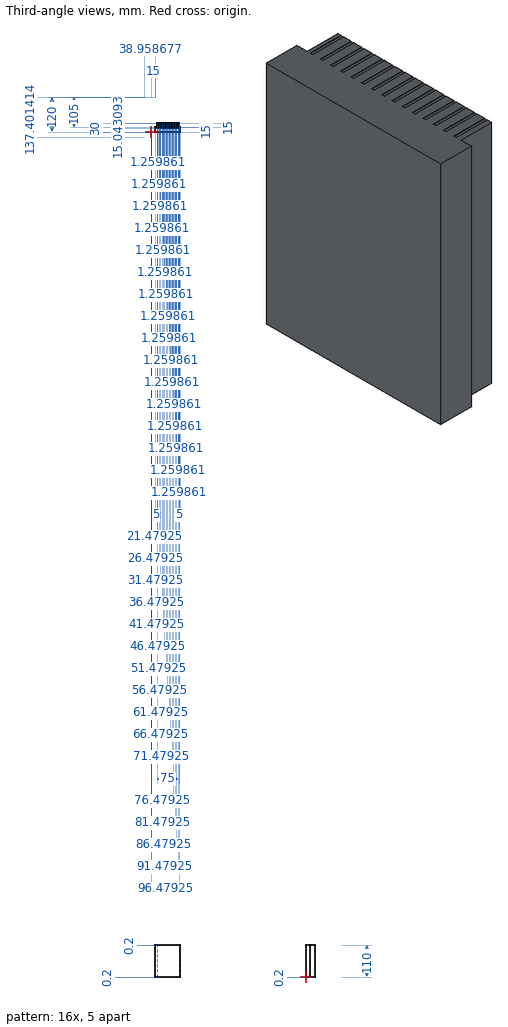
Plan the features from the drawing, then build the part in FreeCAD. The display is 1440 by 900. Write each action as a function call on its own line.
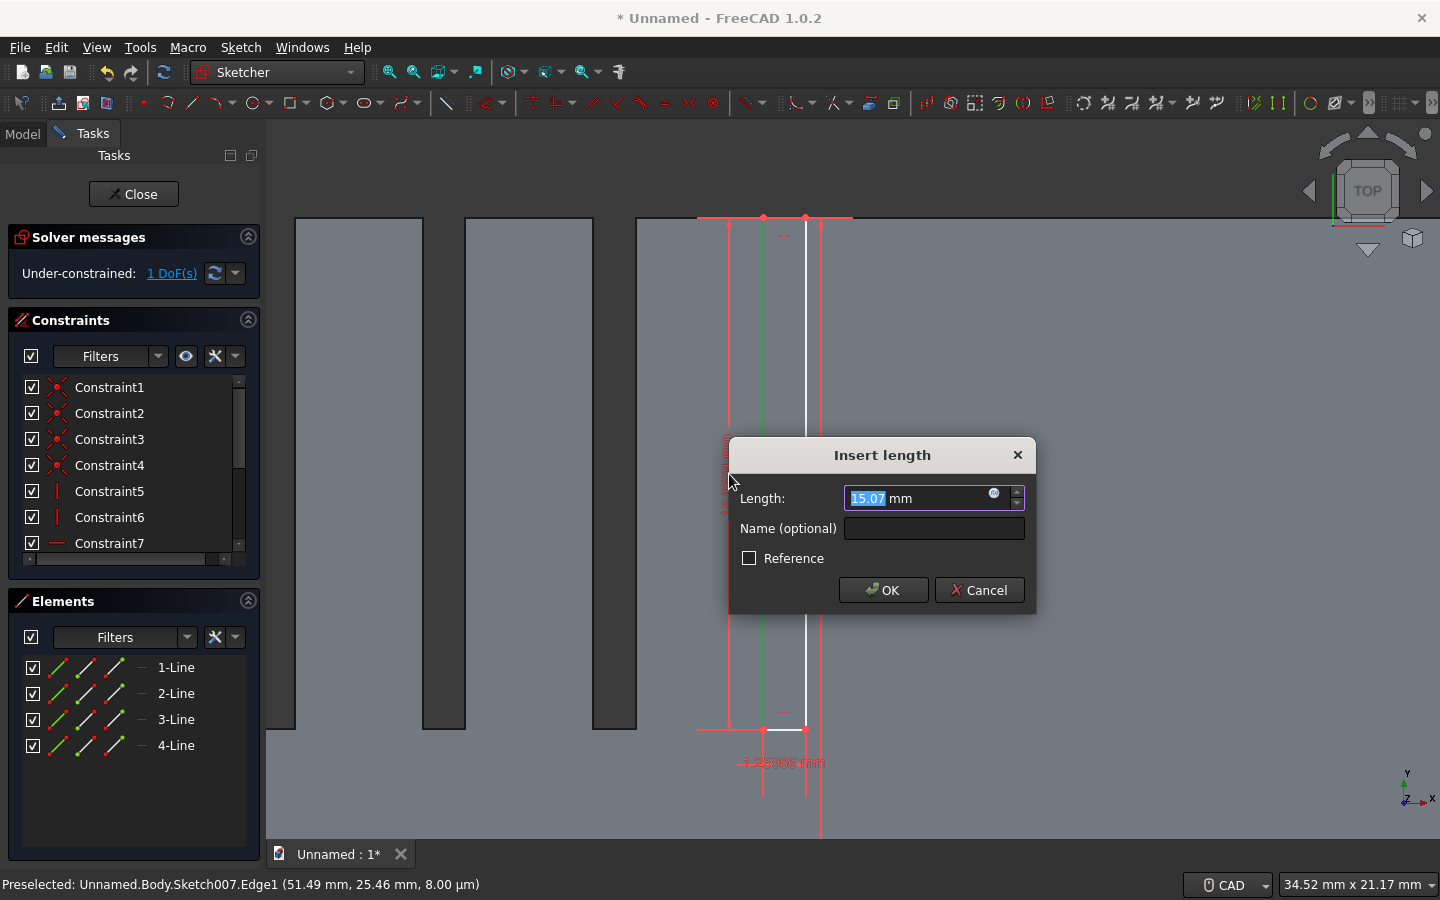
text(15.043093)
key(Return)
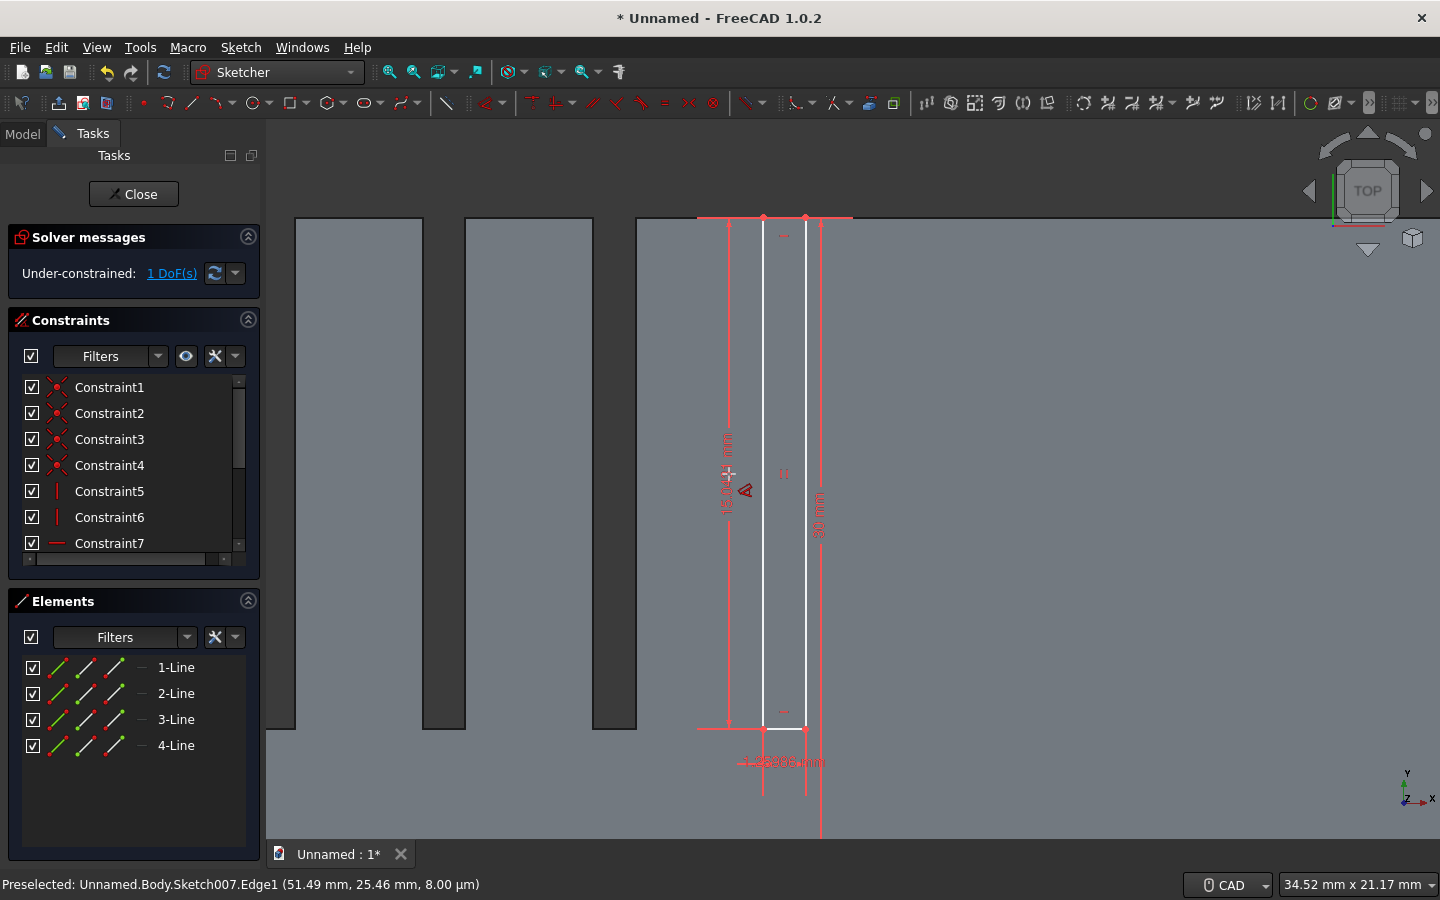
click(763, 218)
click(529, 184)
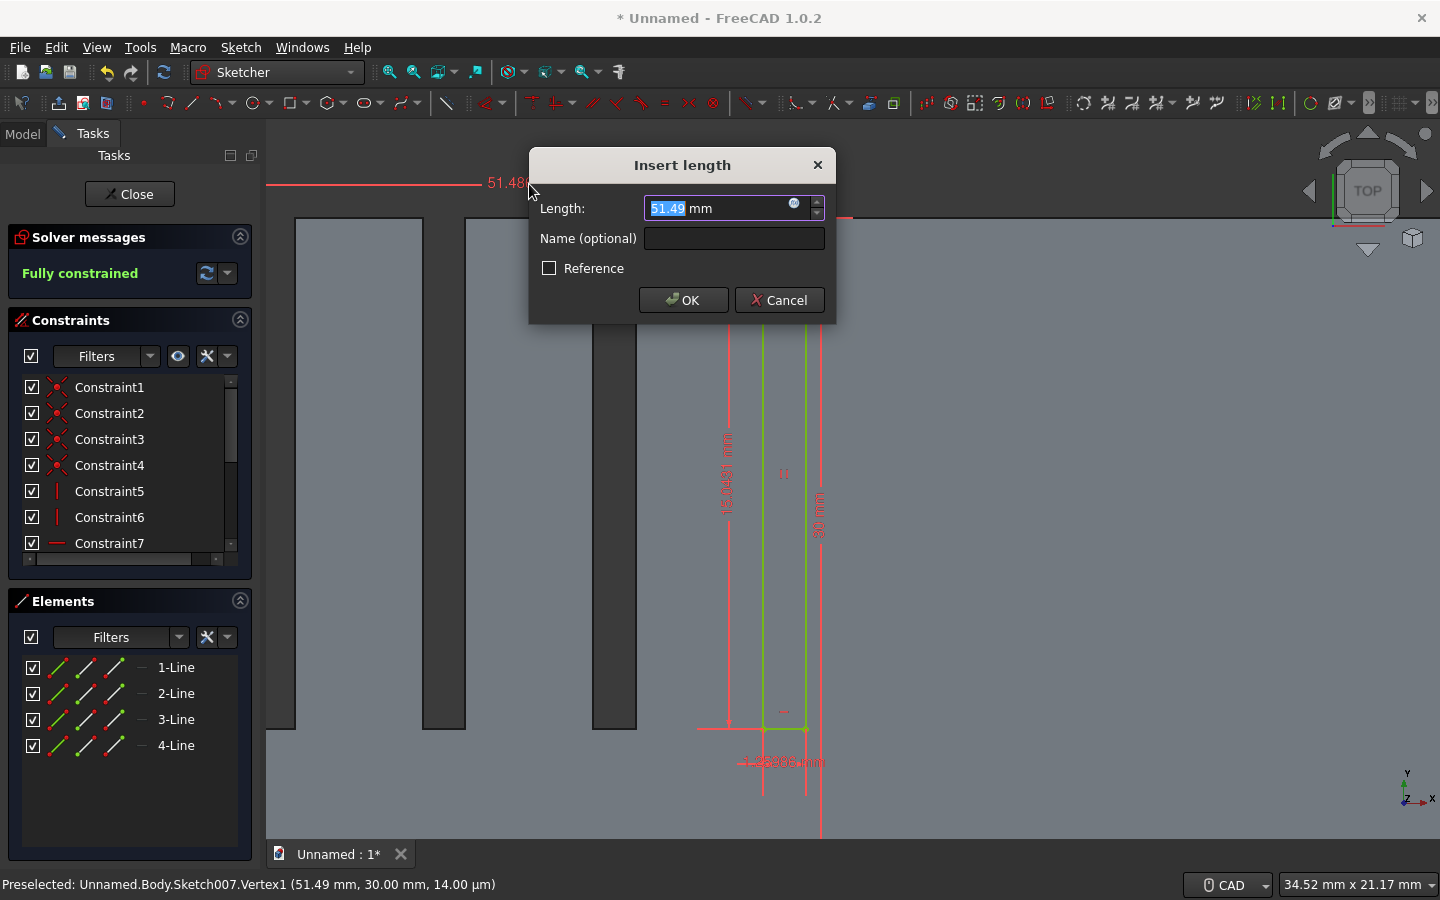
text(51.47925)
key(Return)
key(Escape)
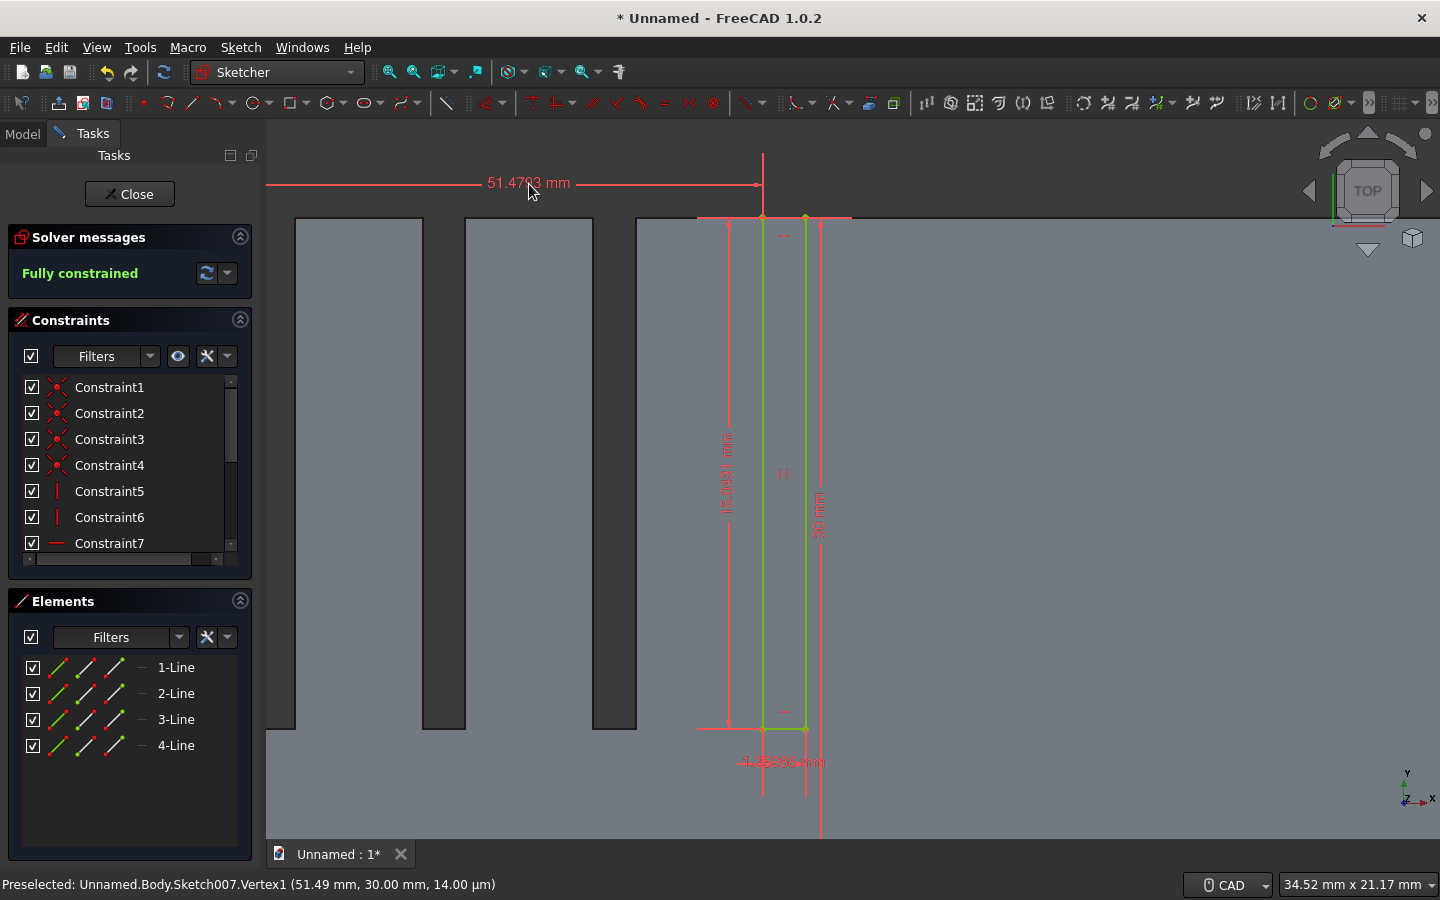
click(130, 194)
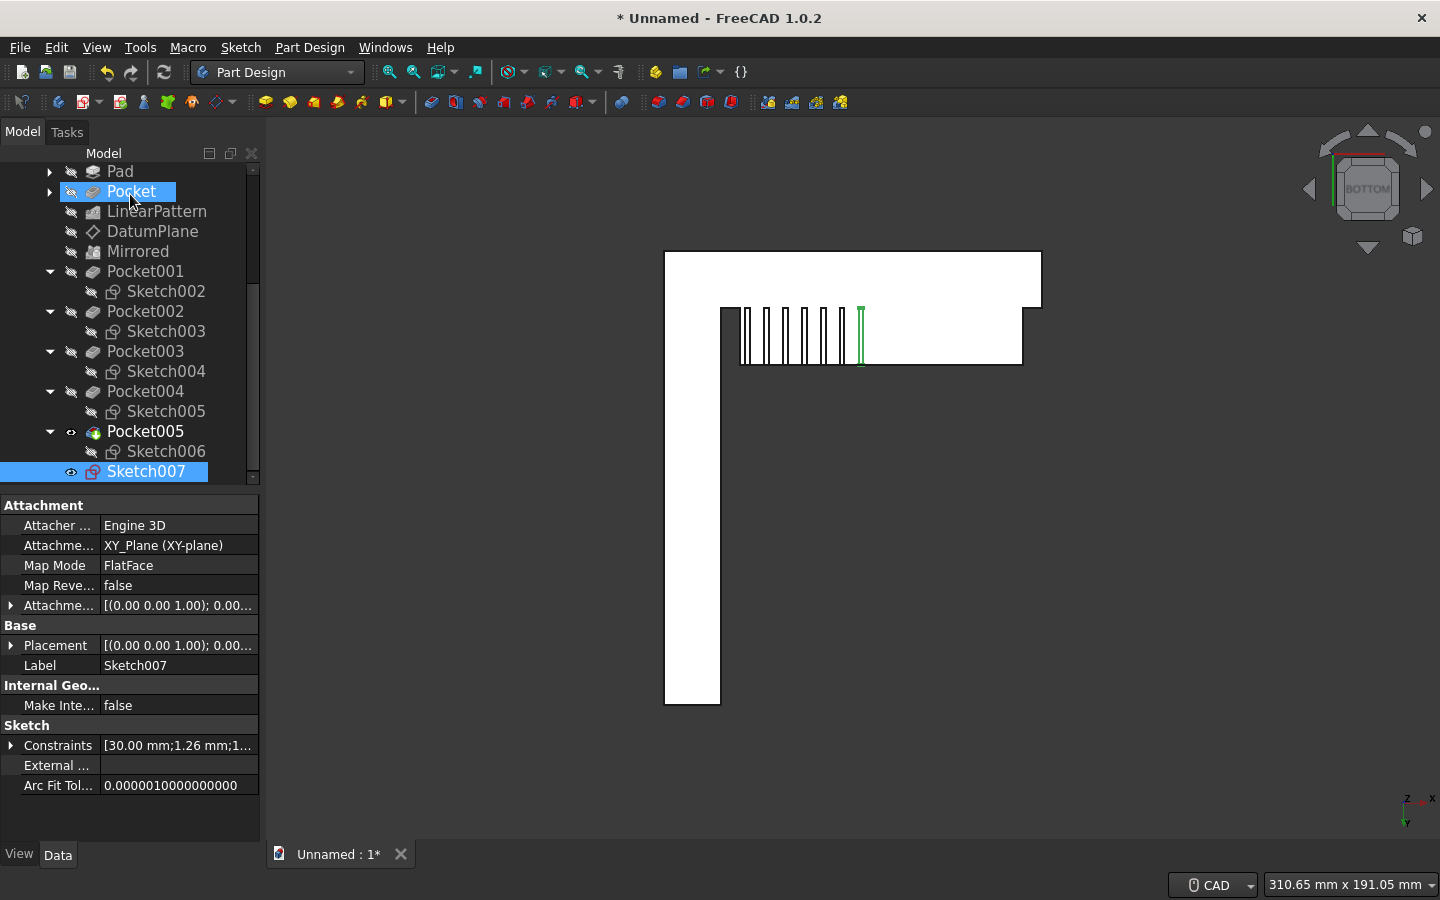
click(432, 102)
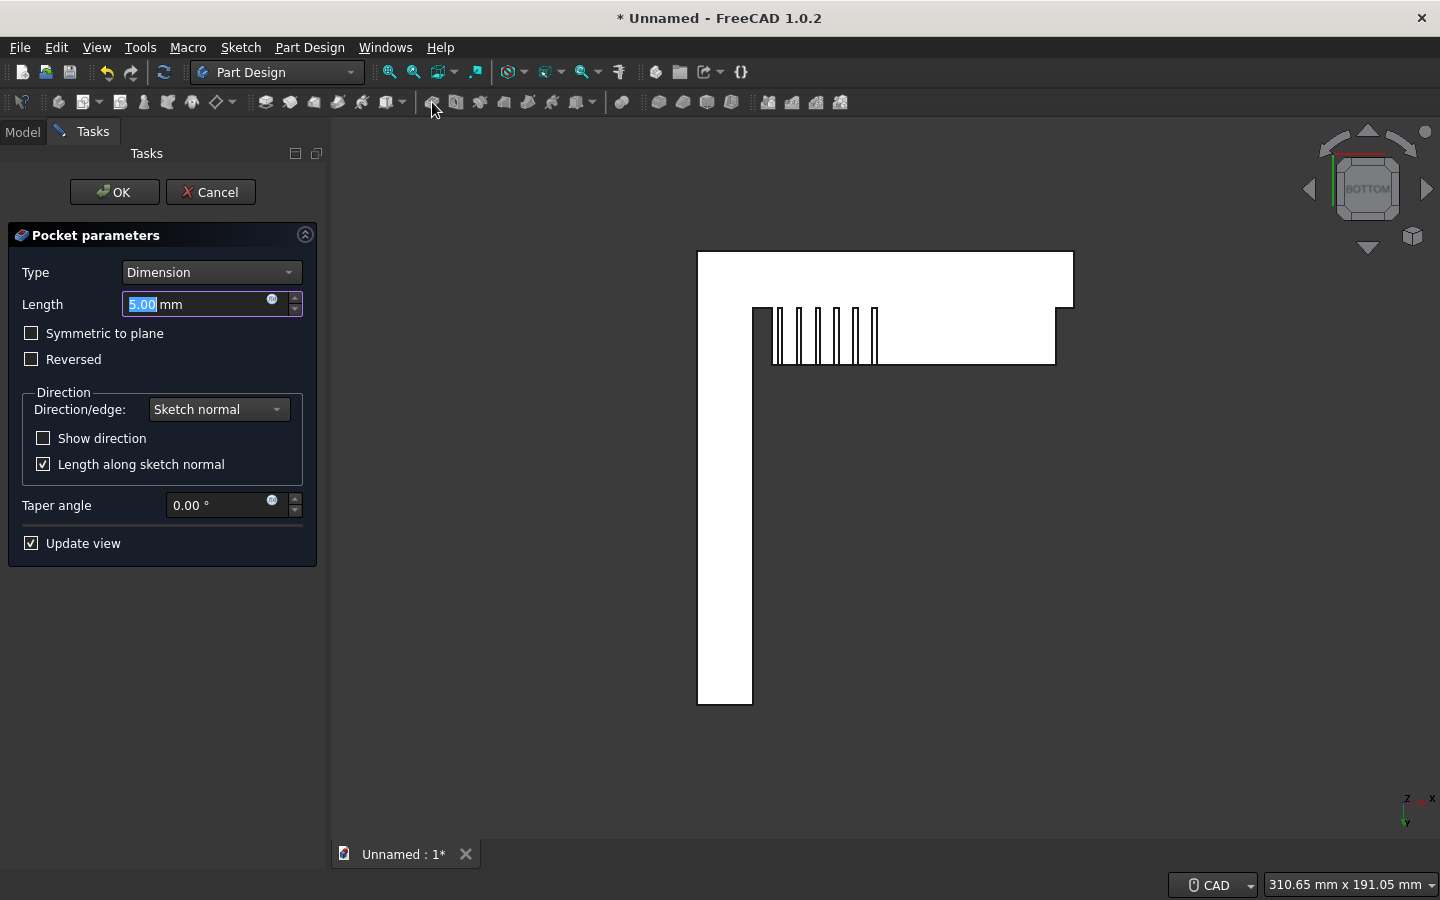
text(0.2)
key(Tab)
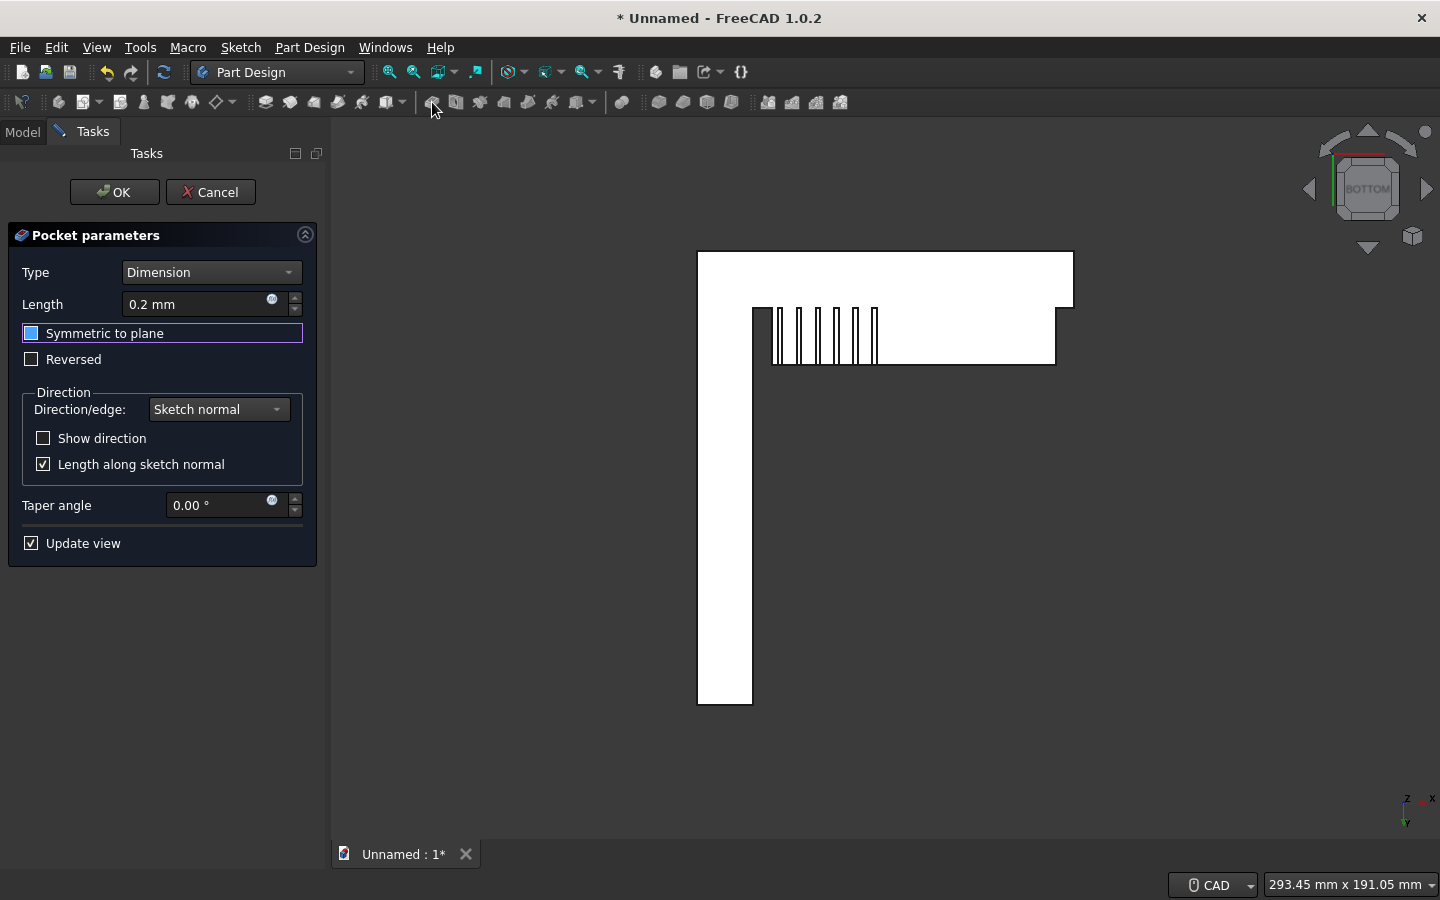
click(30, 359)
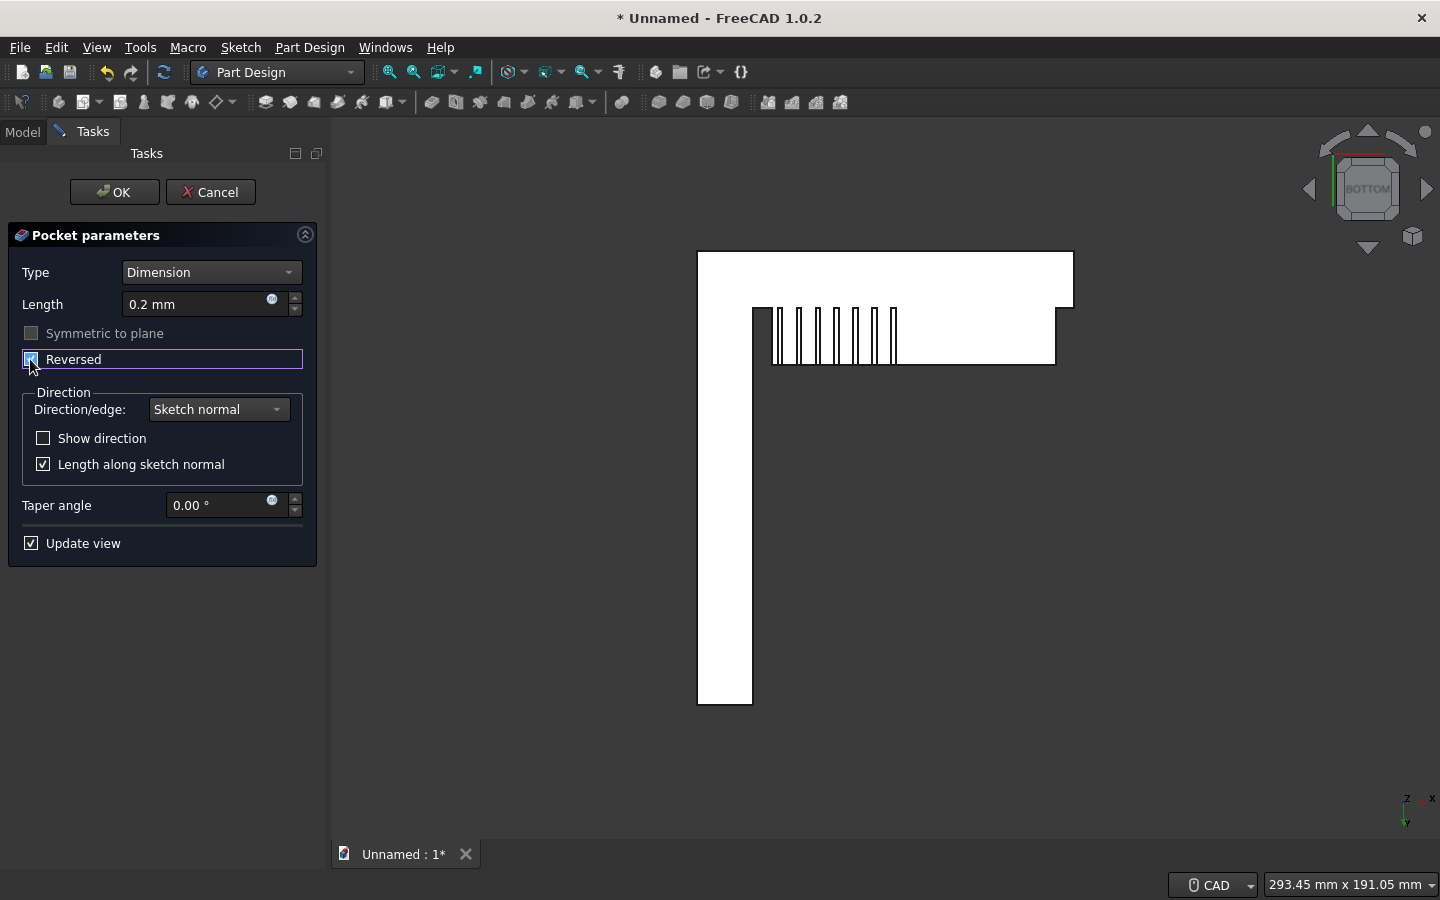
click(115, 192)